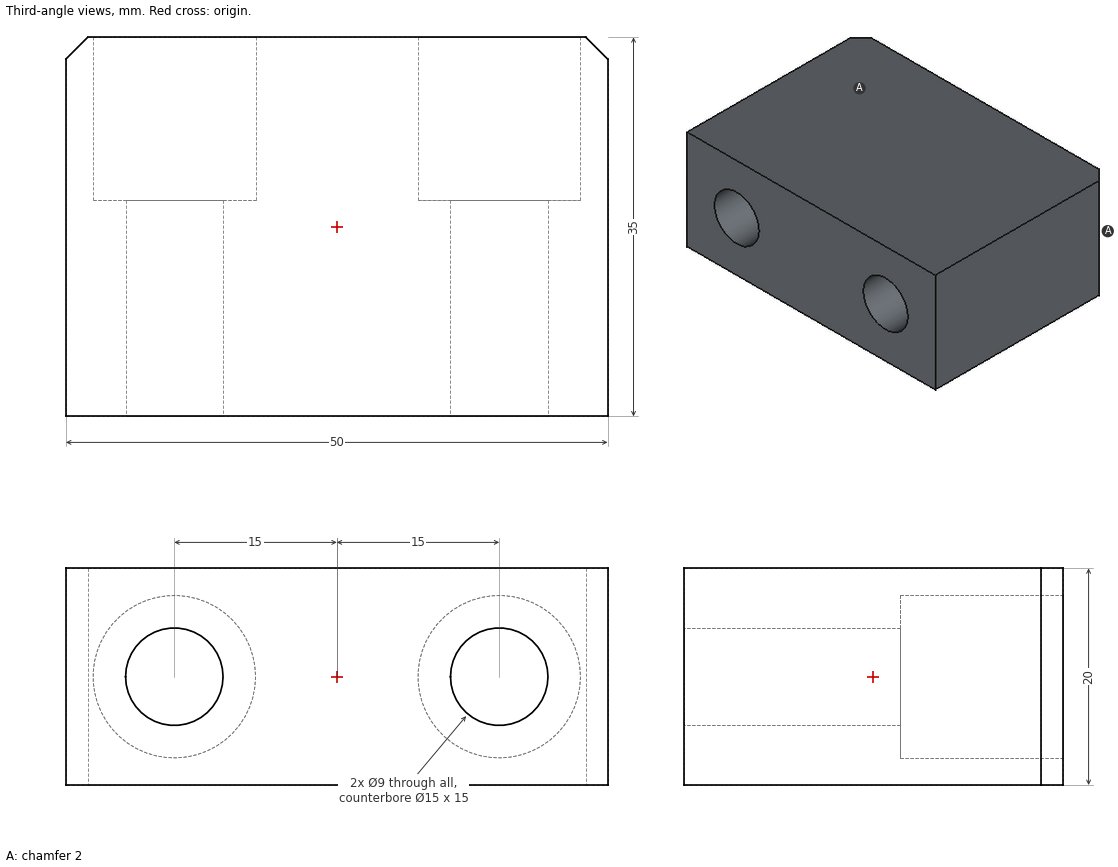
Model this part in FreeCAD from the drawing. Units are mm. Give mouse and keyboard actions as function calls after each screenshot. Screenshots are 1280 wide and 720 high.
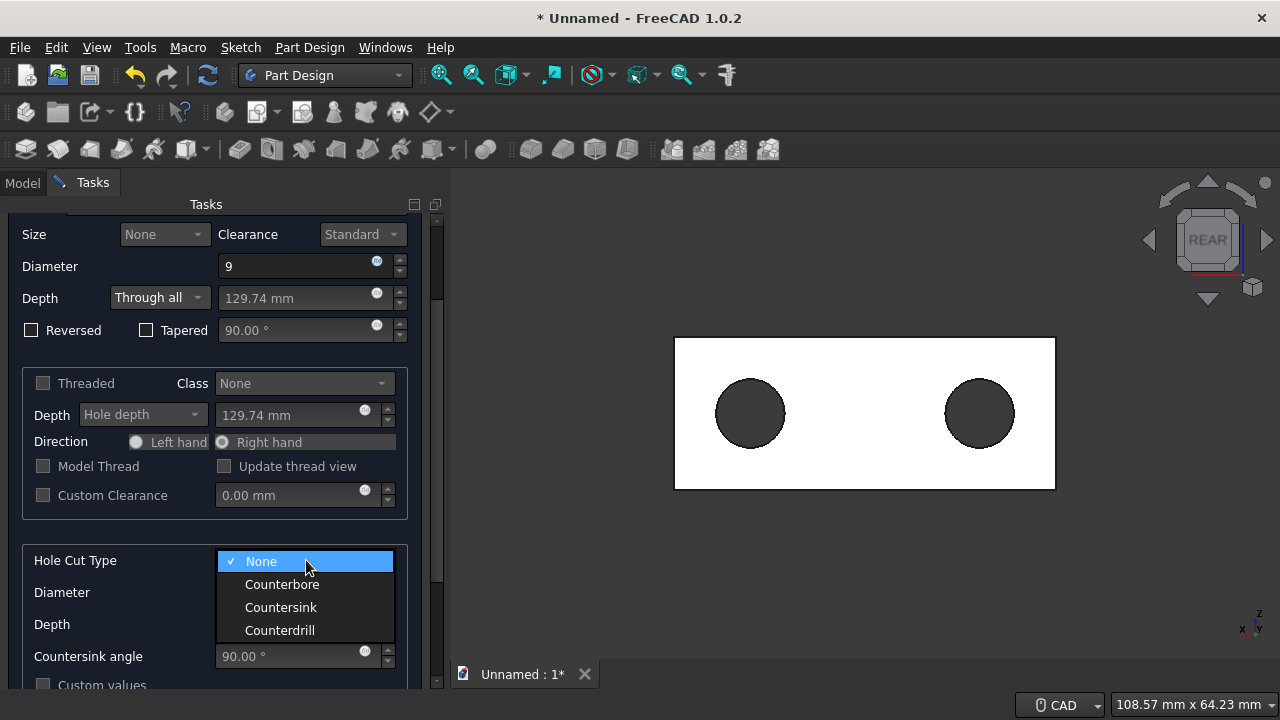
click(304, 584)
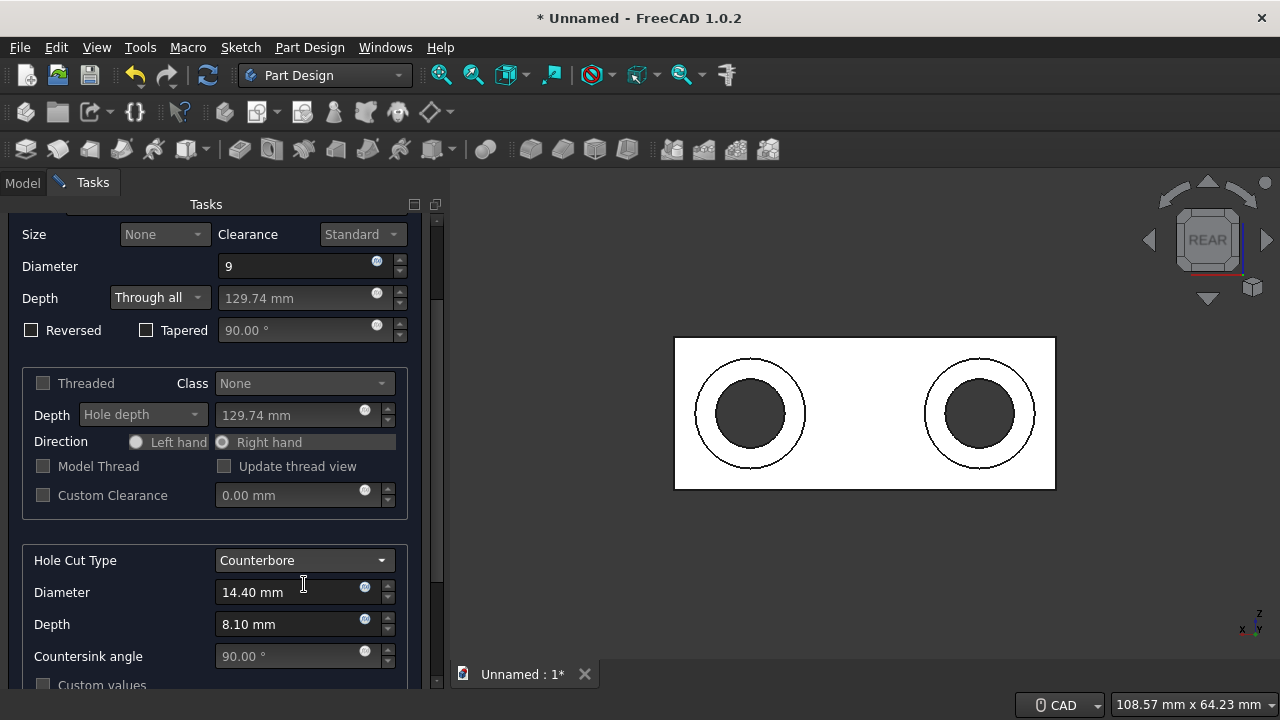
triple_click(298, 592)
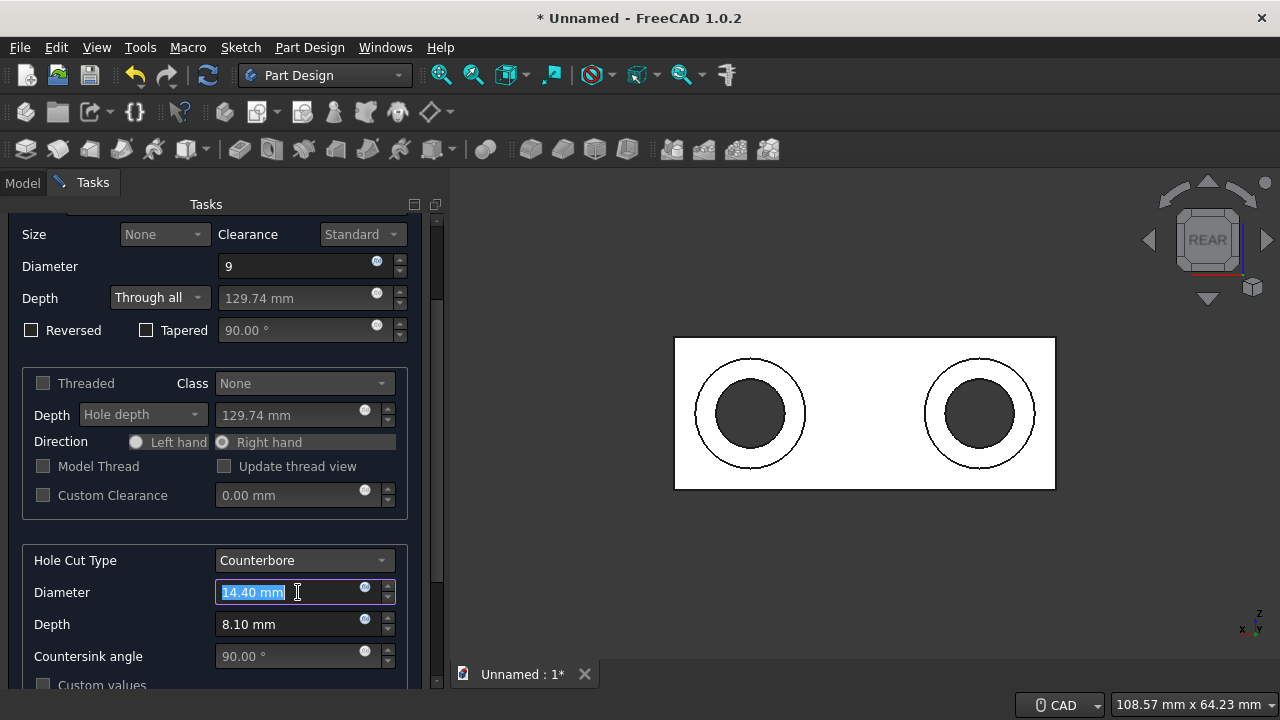
text(15)
key(Tab)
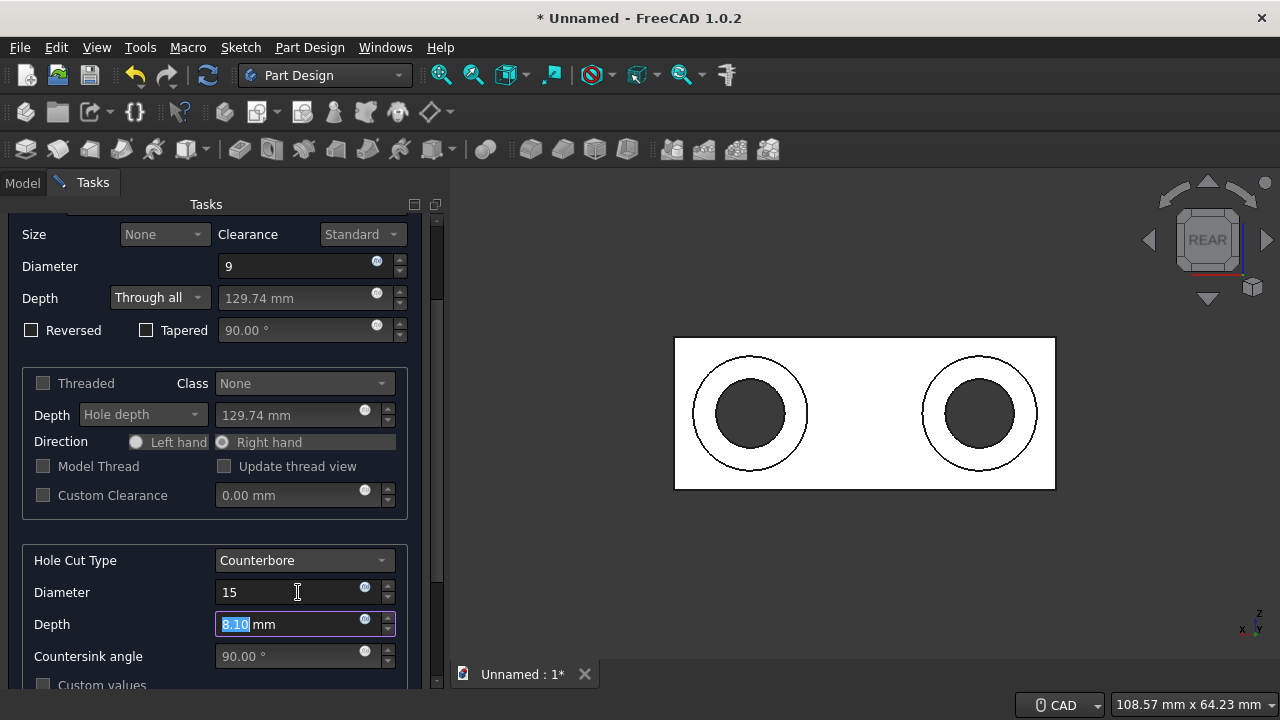
text(15)
key(Tab)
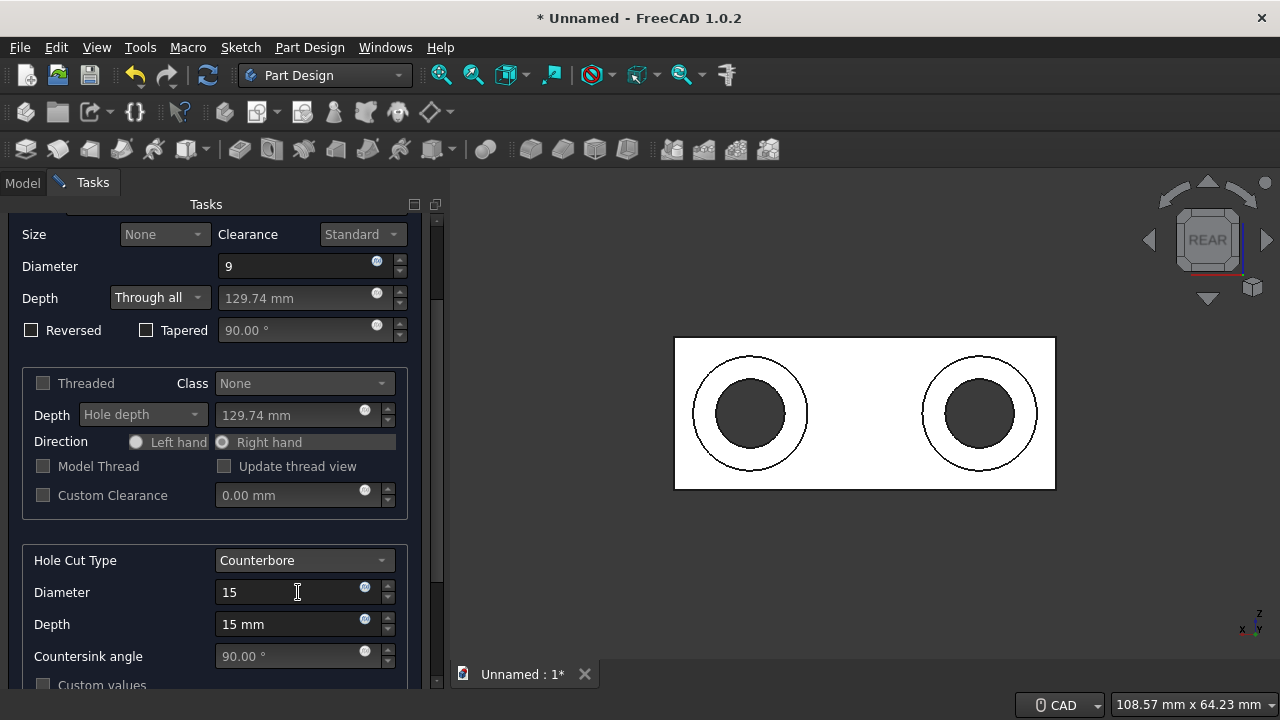
scroll(437, 451, up, 3)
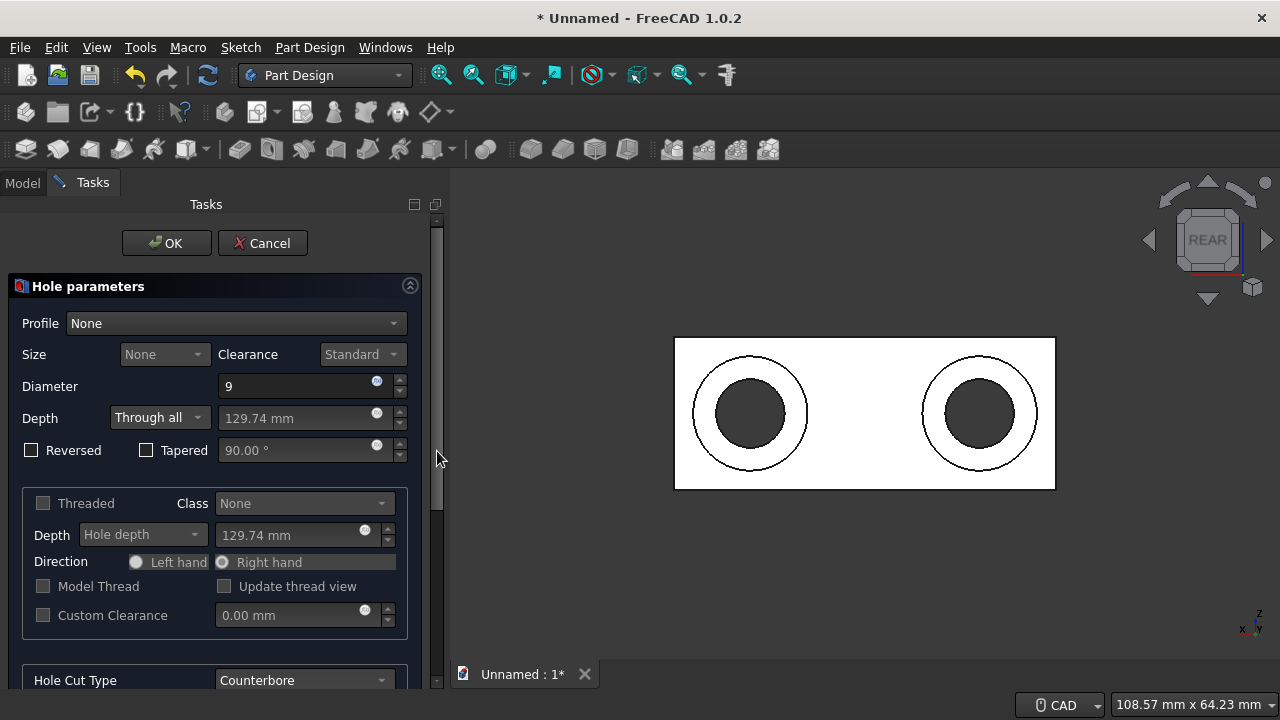
click(167, 243)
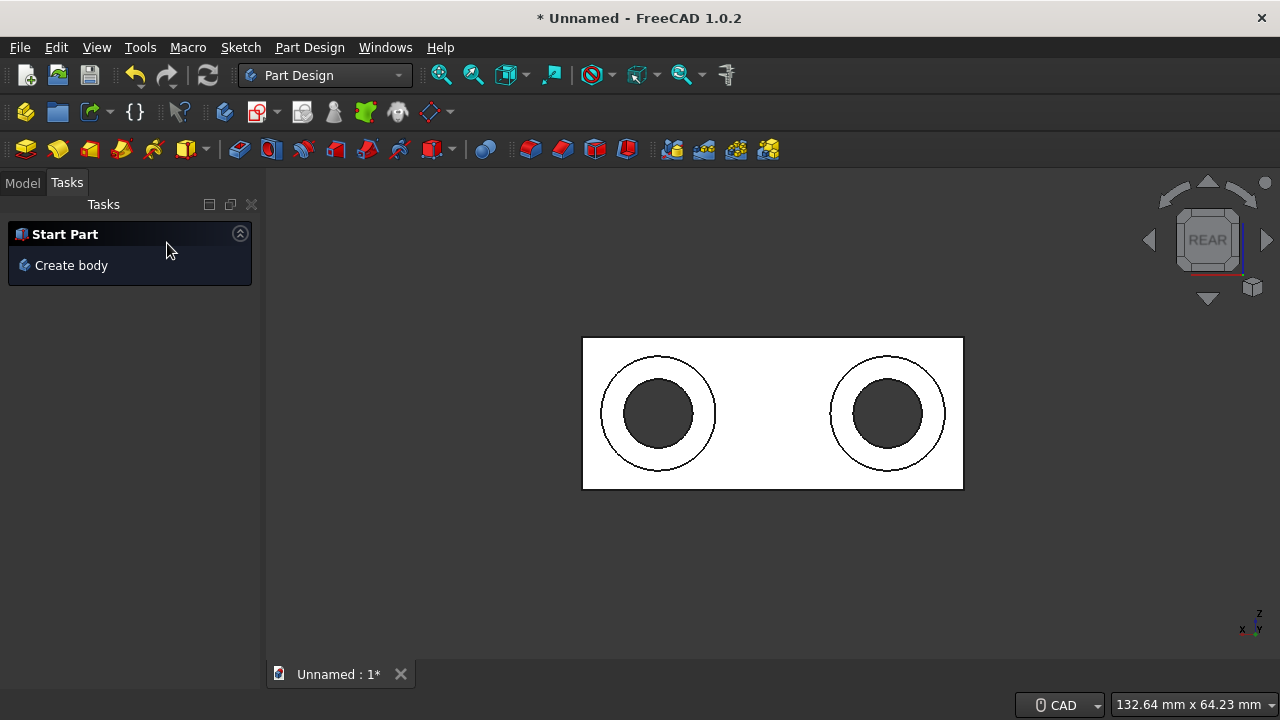
click(442, 76)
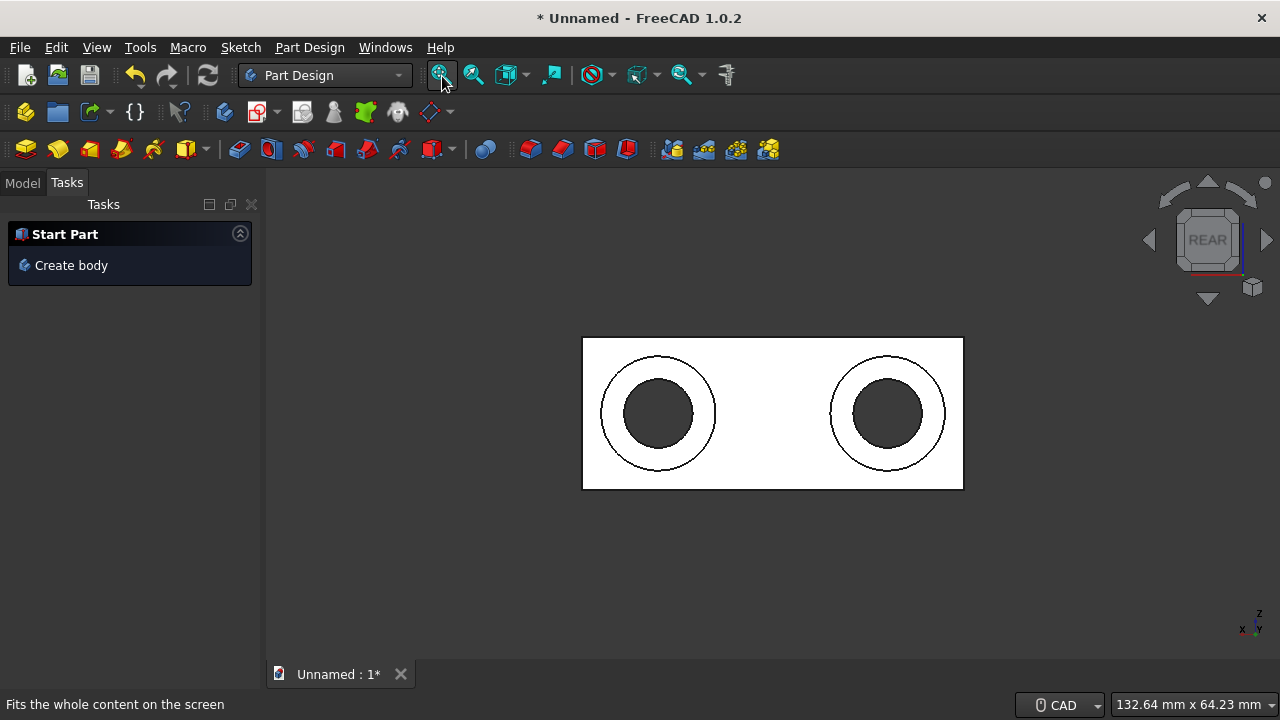
click(964, 412)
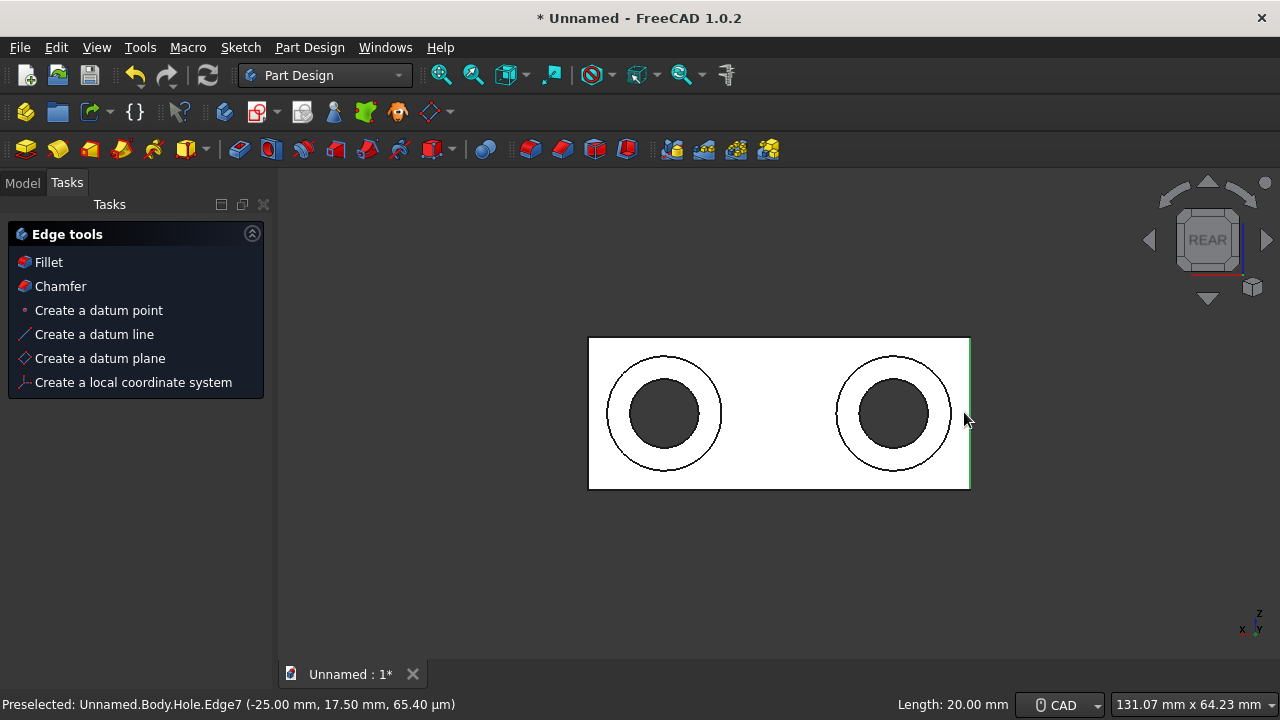
key(0)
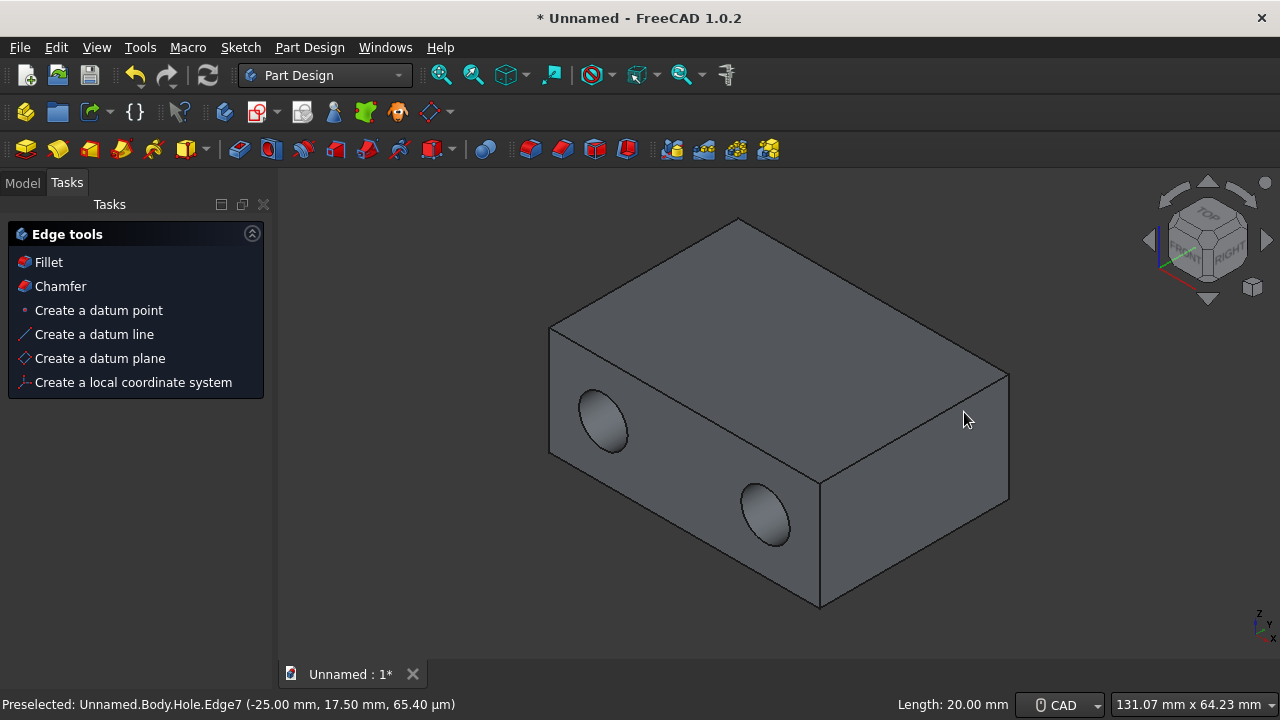
key(2)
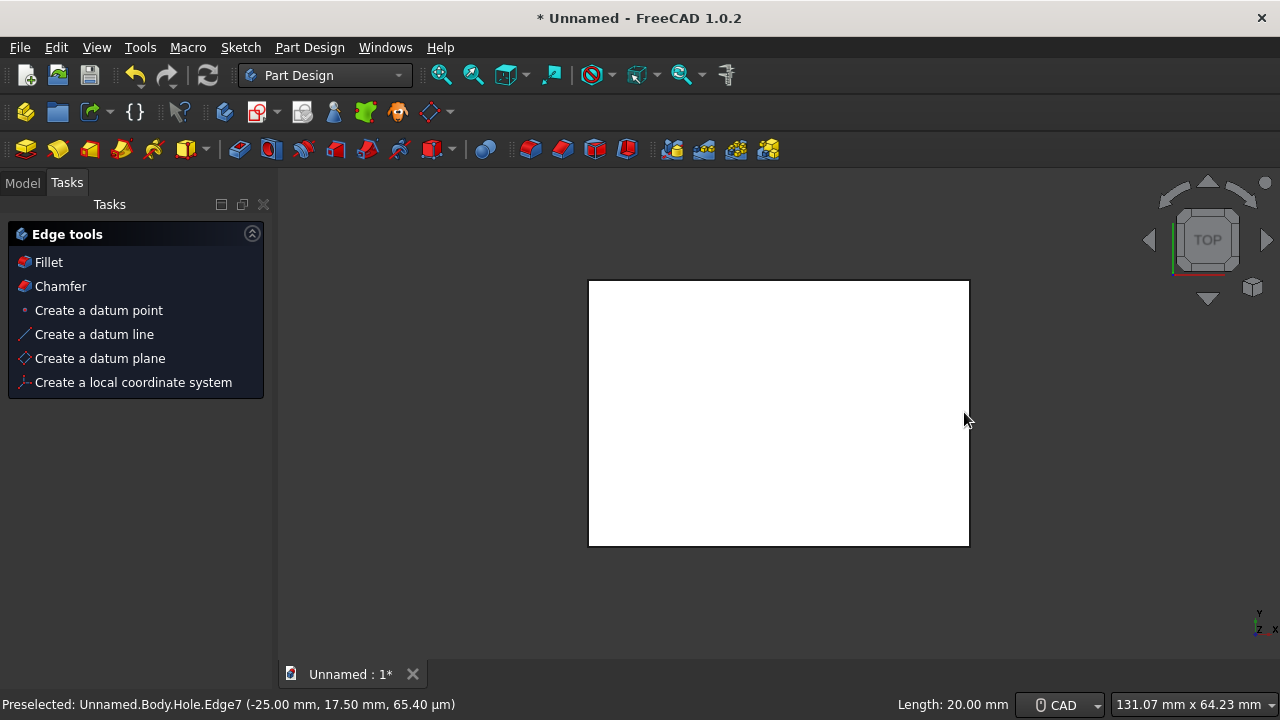
key(1)